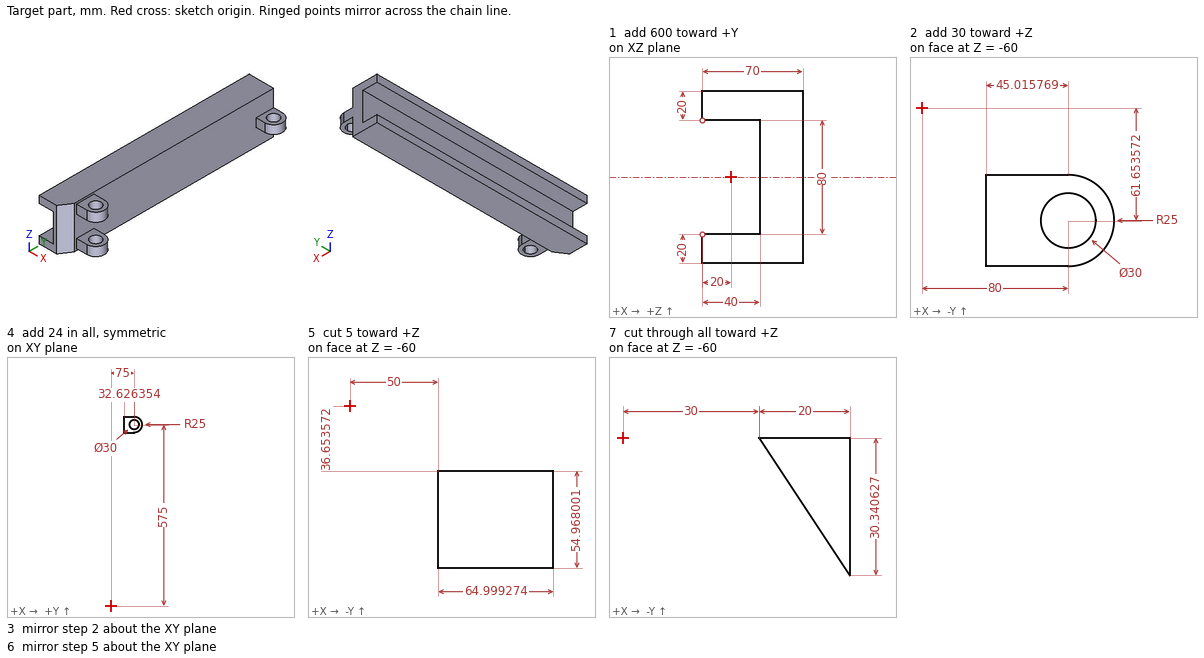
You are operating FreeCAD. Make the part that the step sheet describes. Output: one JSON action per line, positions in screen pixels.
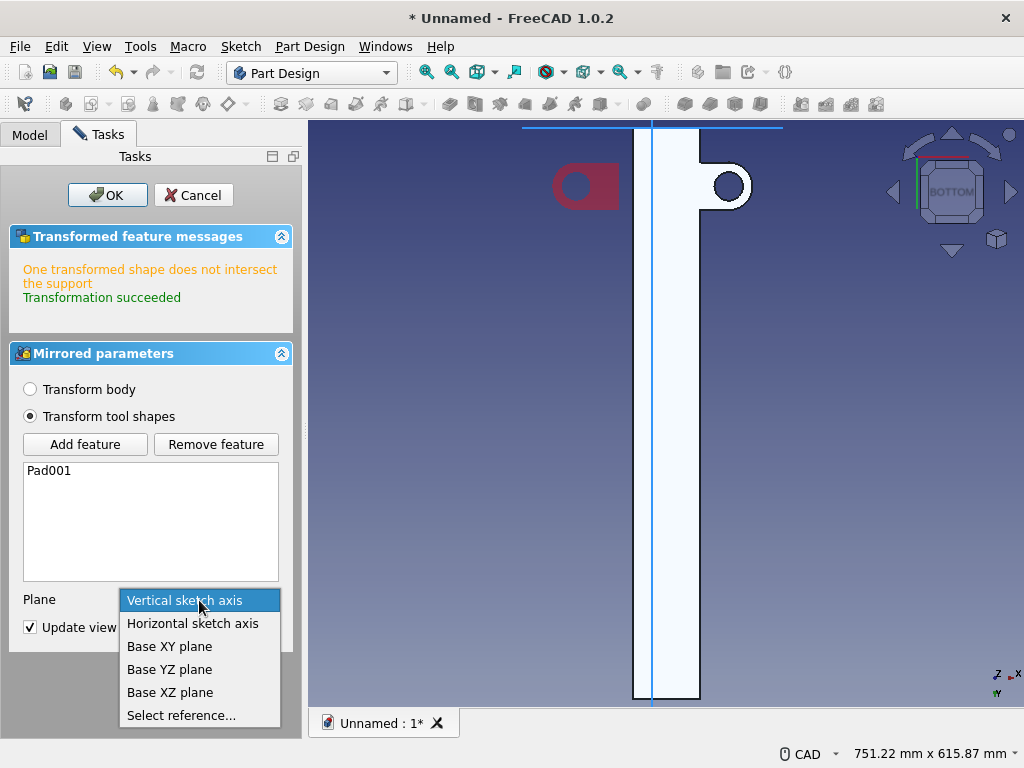
{"action": "left_click", "coordinate": [198, 646]}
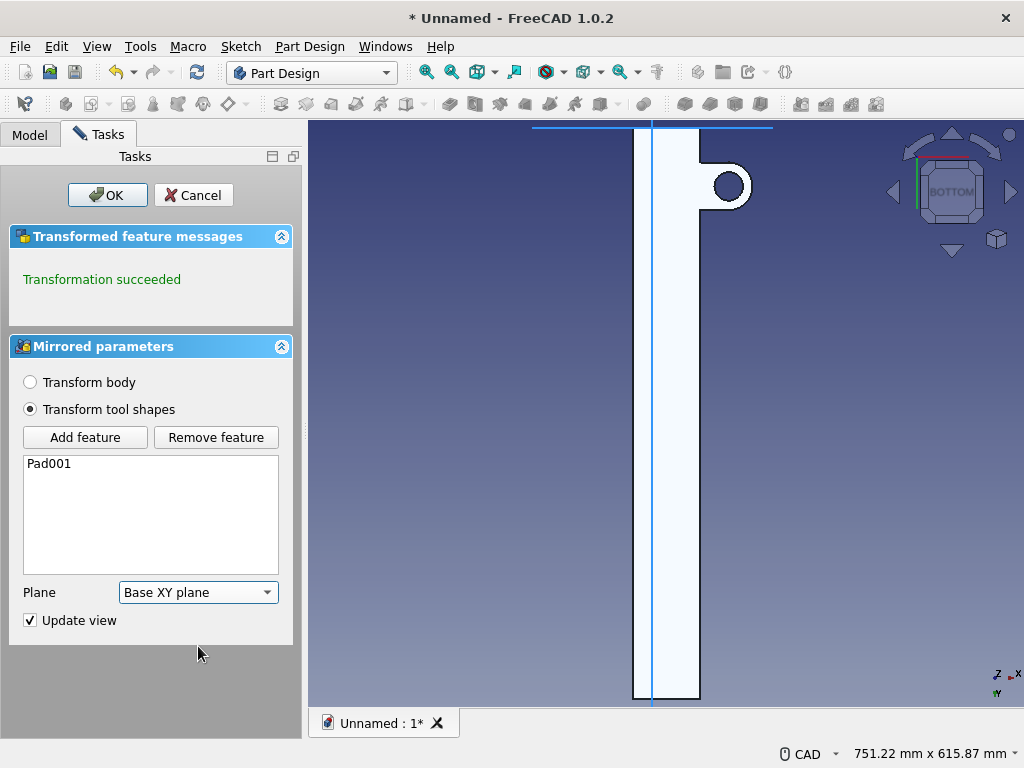
{"action": "left_click", "coordinate": [108, 195]}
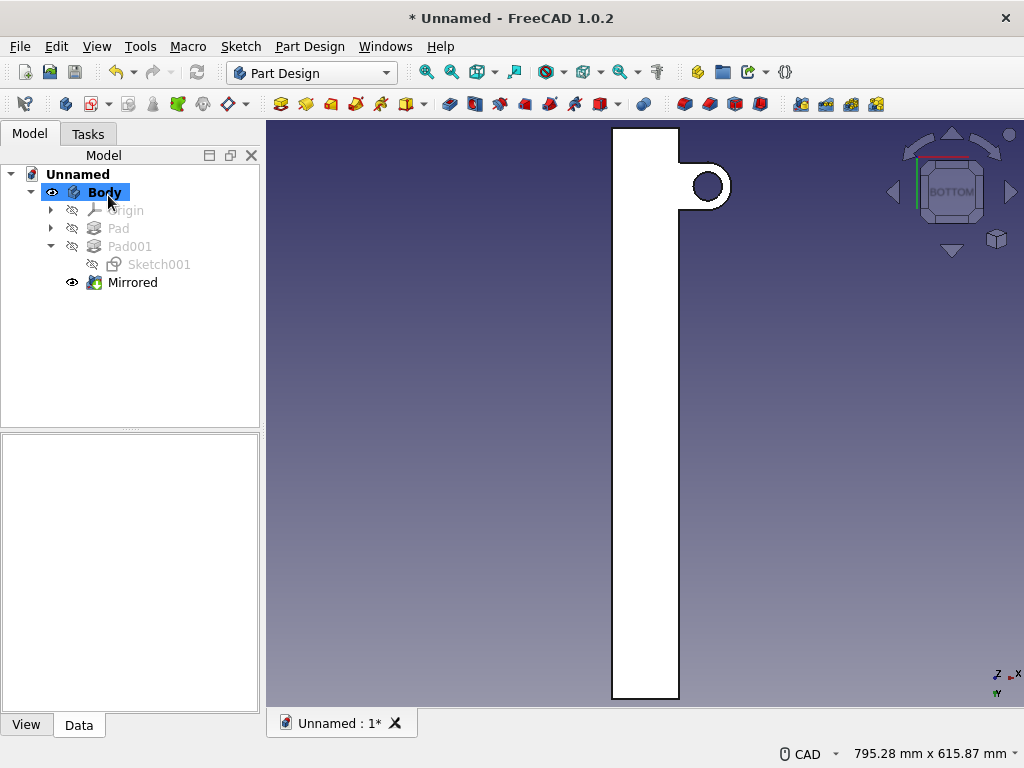
{"action": "left_click", "coordinate": [90, 104]}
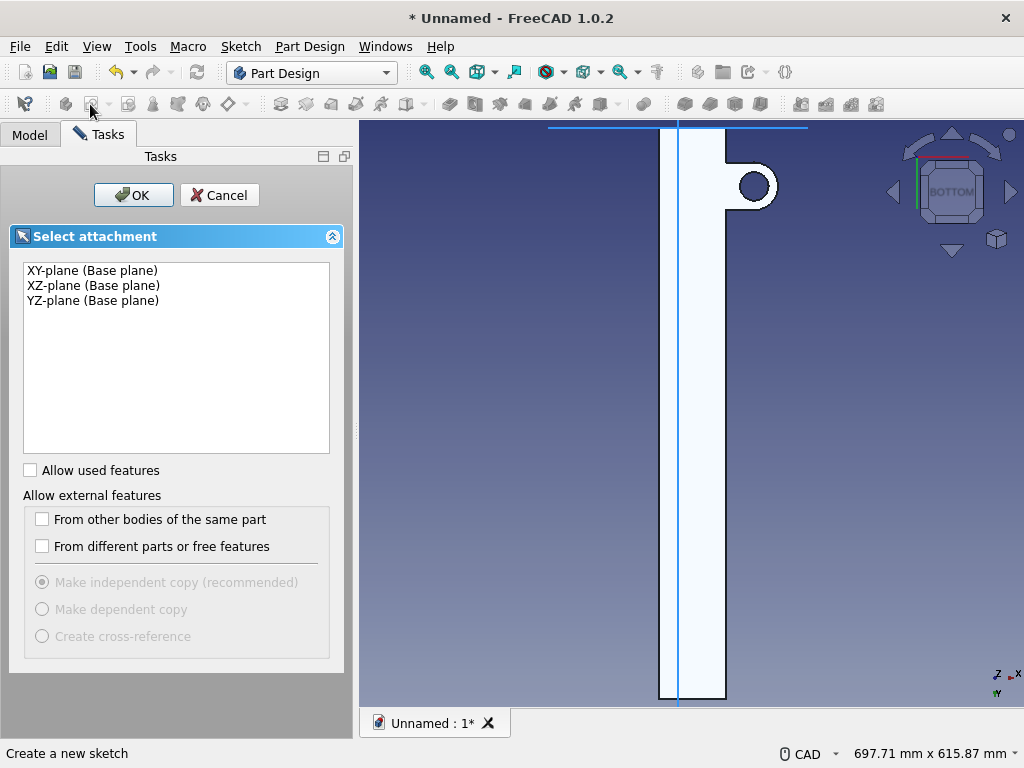
{"action": "left_click", "coordinate": [84, 270]}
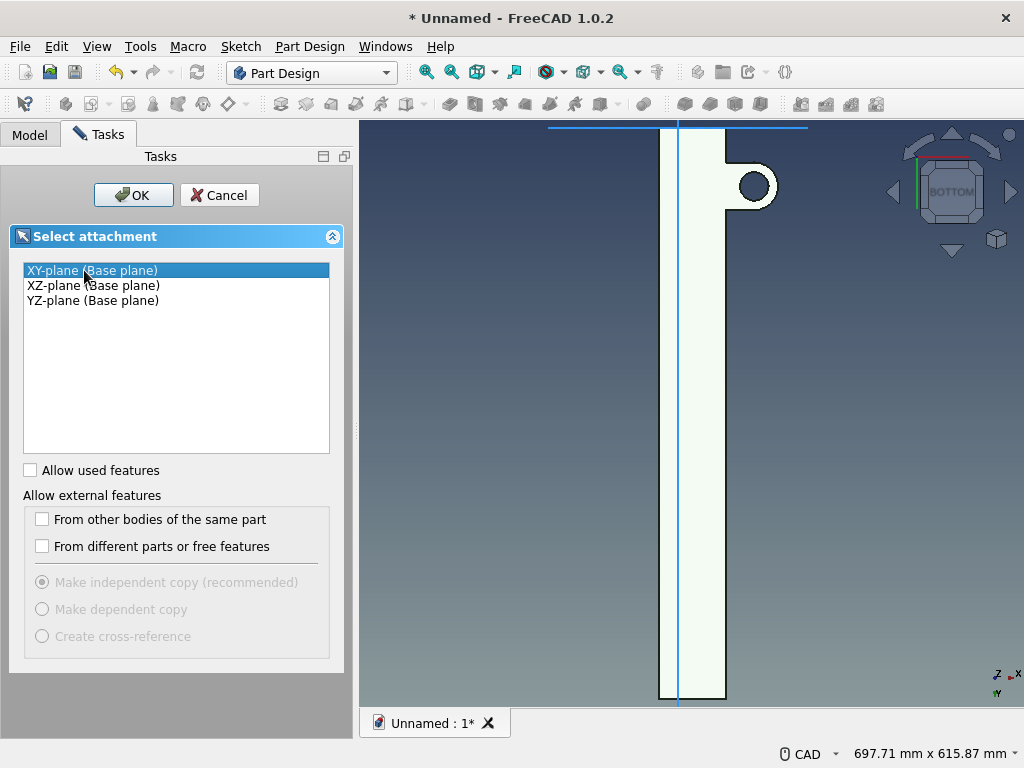
{"action": "left_click", "coordinate": [134, 195]}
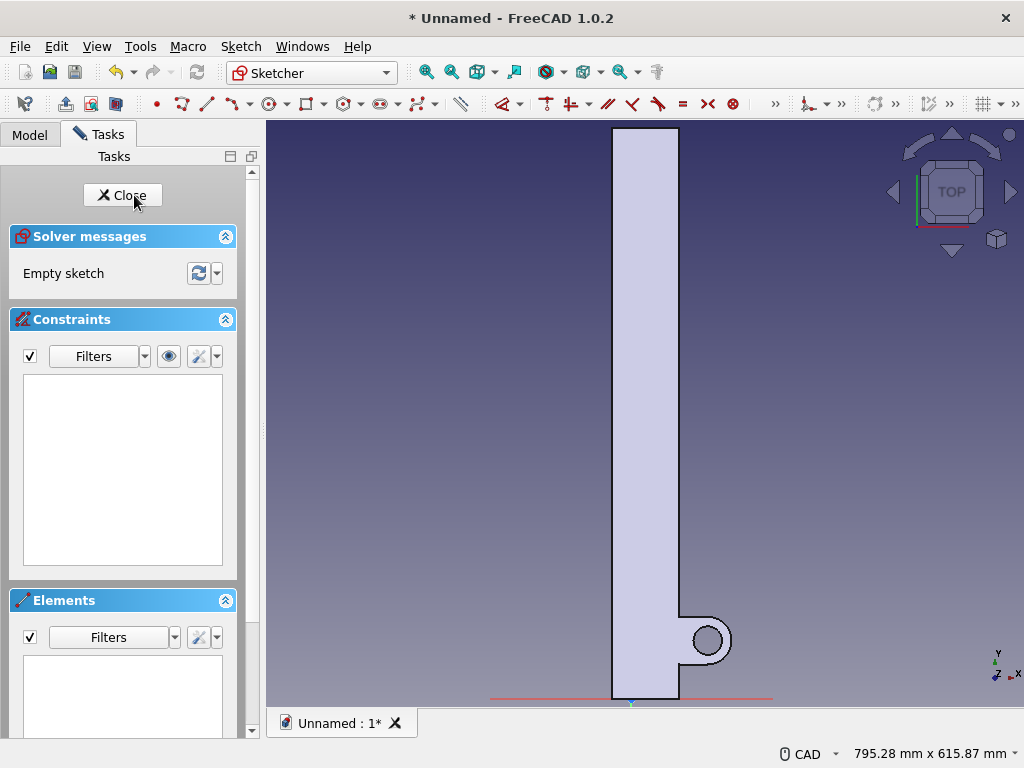
{"action": "left_click", "coordinate": [116, 104]}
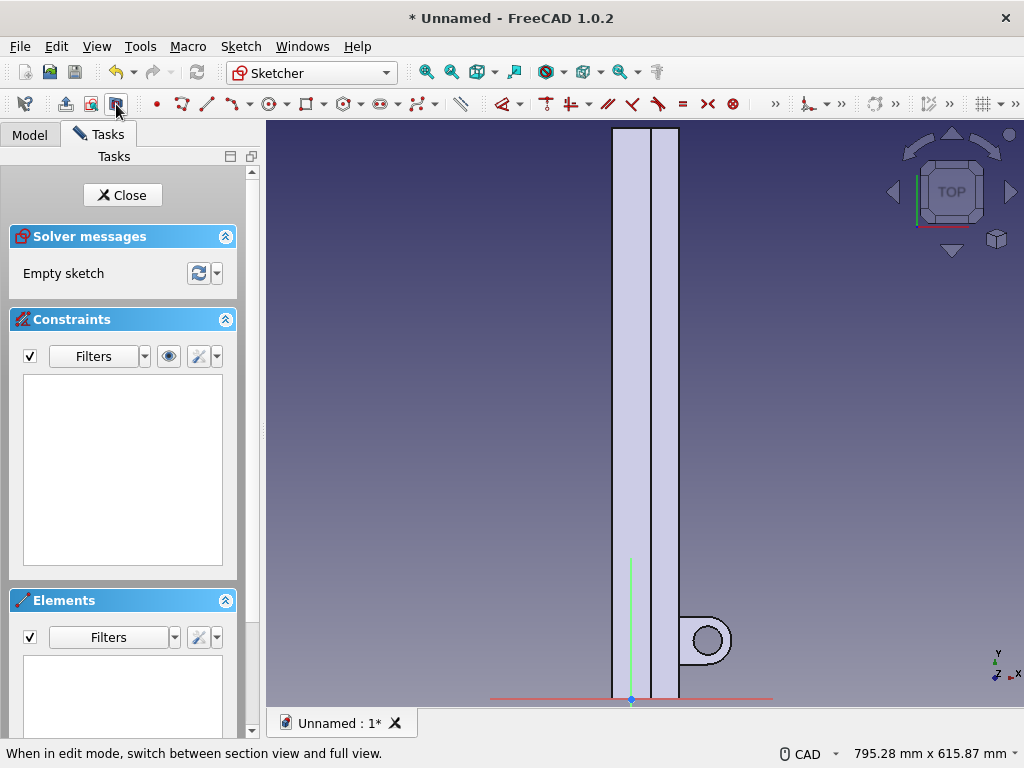
{"action": "scroll", "coordinate": [576, 414], "scroll_direction": "down", "scroll_amount": 5}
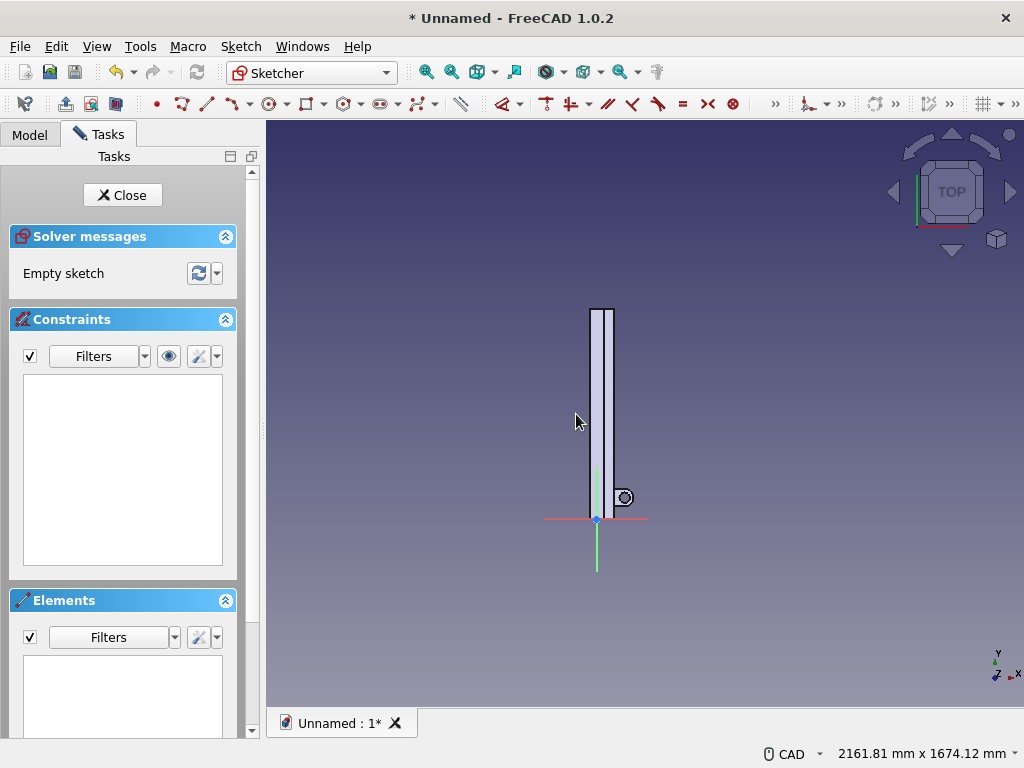
{"action": "scroll", "coordinate": [624, 313], "scroll_direction": "up", "scroll_amount": 15}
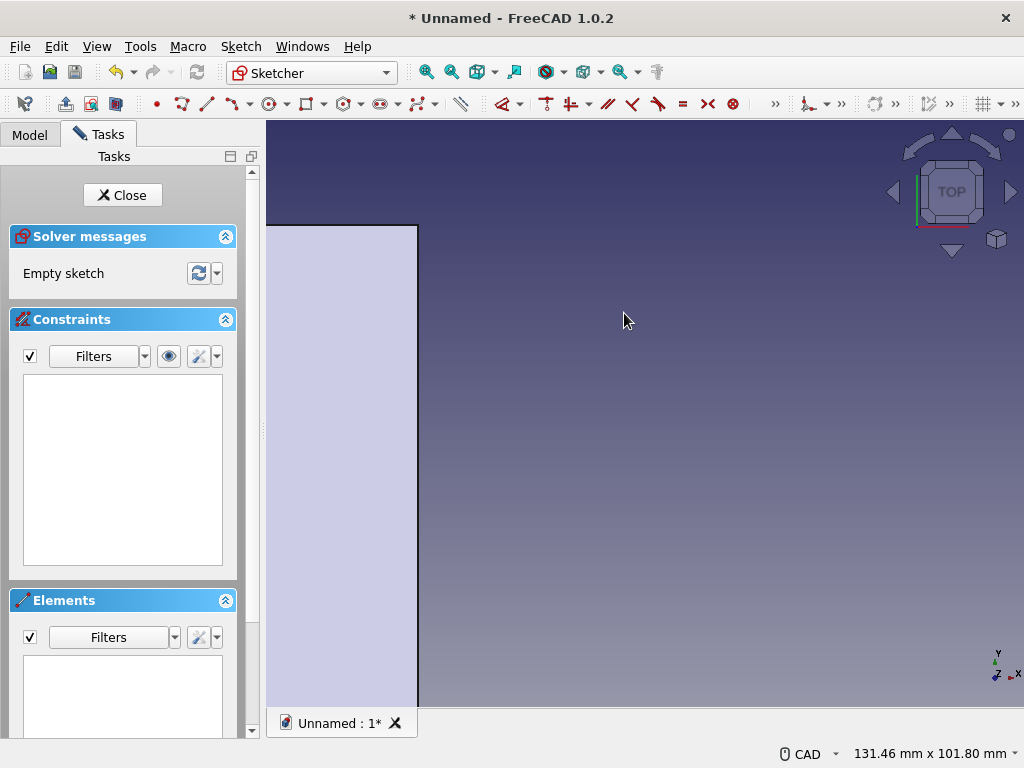
{"action": "left_click", "coordinate": [182, 104]}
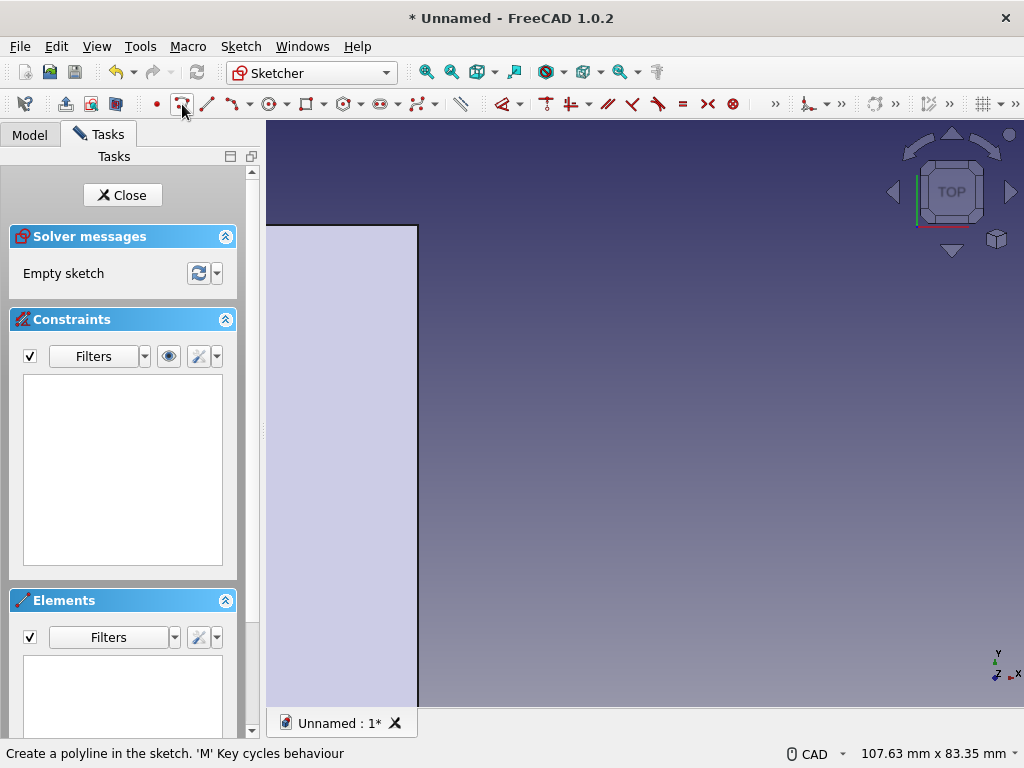
{"action": "left_click", "coordinate": [594, 225]}
{"action": "left_click", "coordinate": [364, 225]}
{"action": "left_click", "coordinate": [364, 577]}
{"action": "left_click", "coordinate": [594, 577]}
{"action": "right_click", "coordinate": [594, 577]}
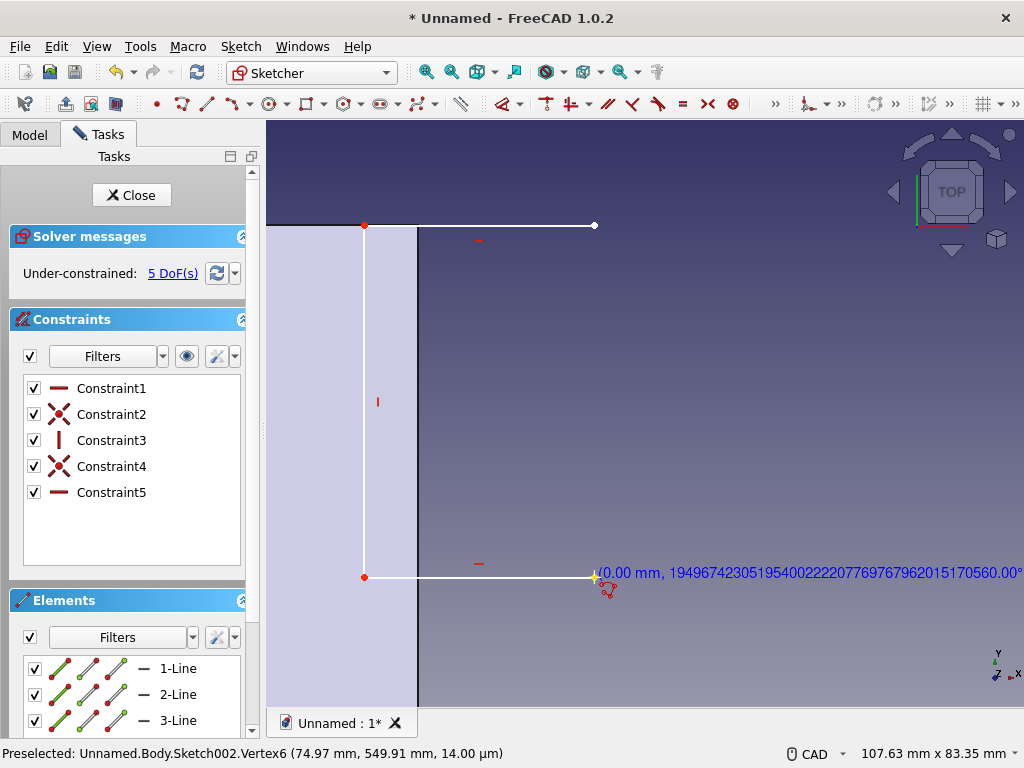
{"action": "left_click", "coordinate": [232, 104]}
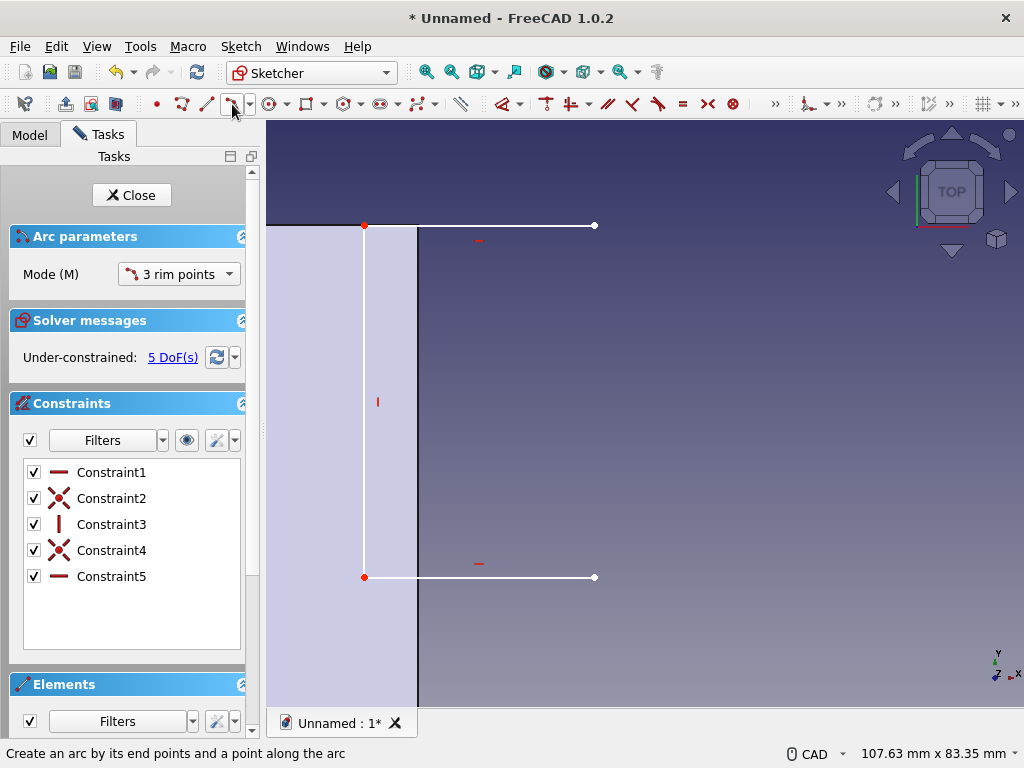
{"action": "left_click", "coordinate": [594, 578]}
{"action": "left_click", "coordinate": [594, 226]}
{"action": "left_click", "coordinate": [770, 401]}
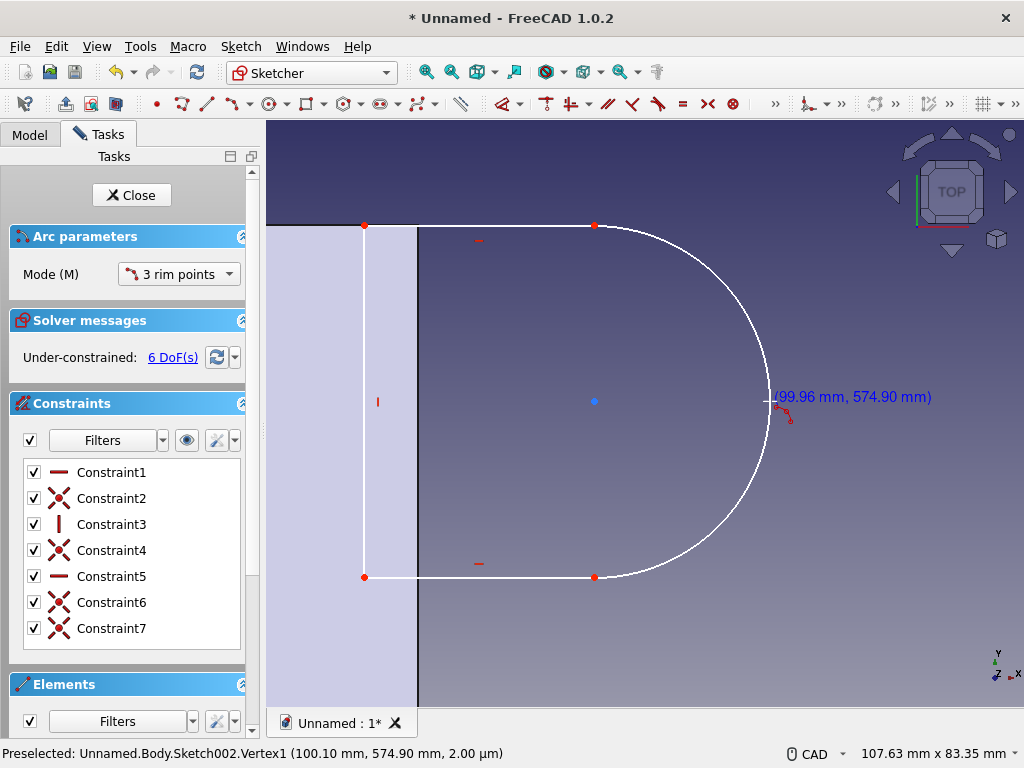
{"action": "left_click", "coordinate": [268, 104]}